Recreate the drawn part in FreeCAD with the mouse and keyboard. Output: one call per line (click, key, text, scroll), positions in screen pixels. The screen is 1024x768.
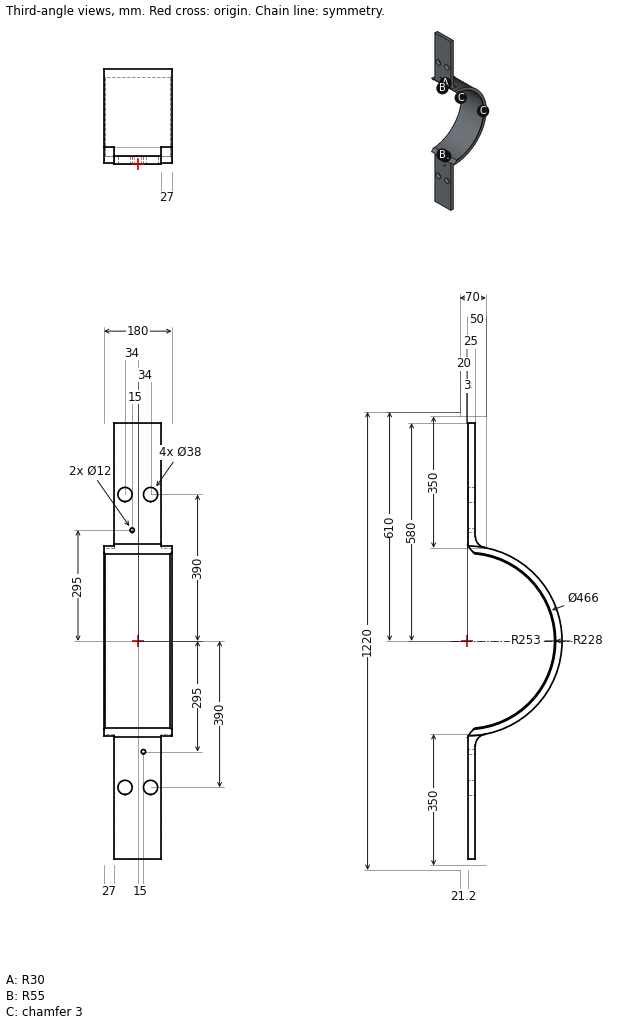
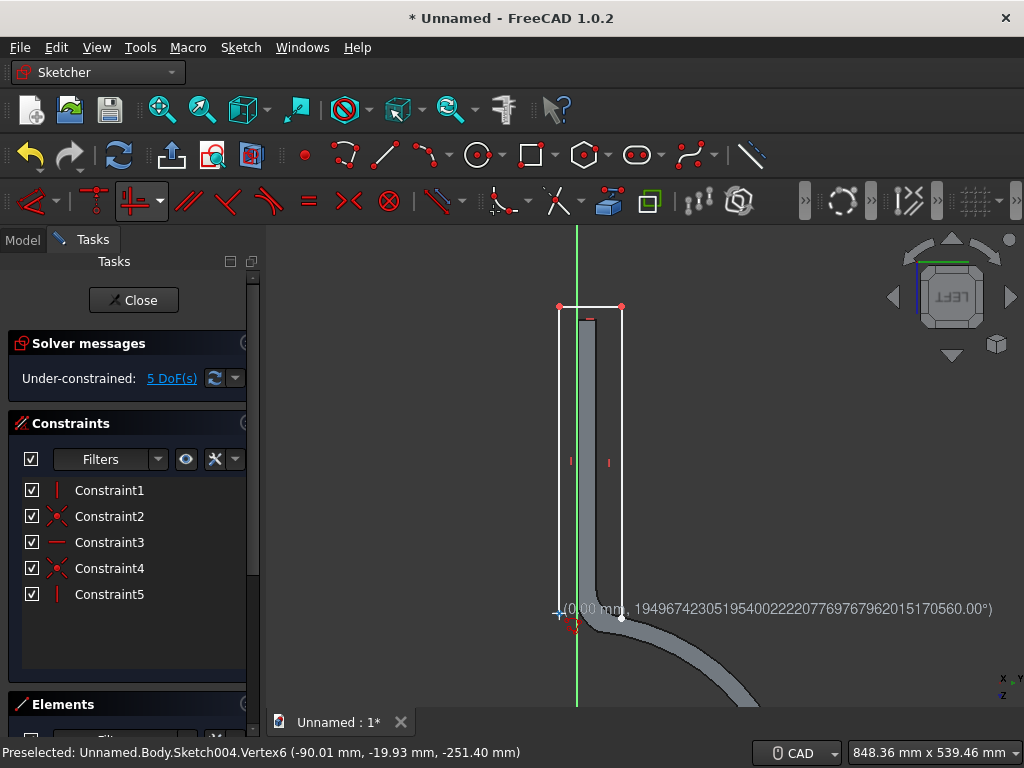
click(426, 156)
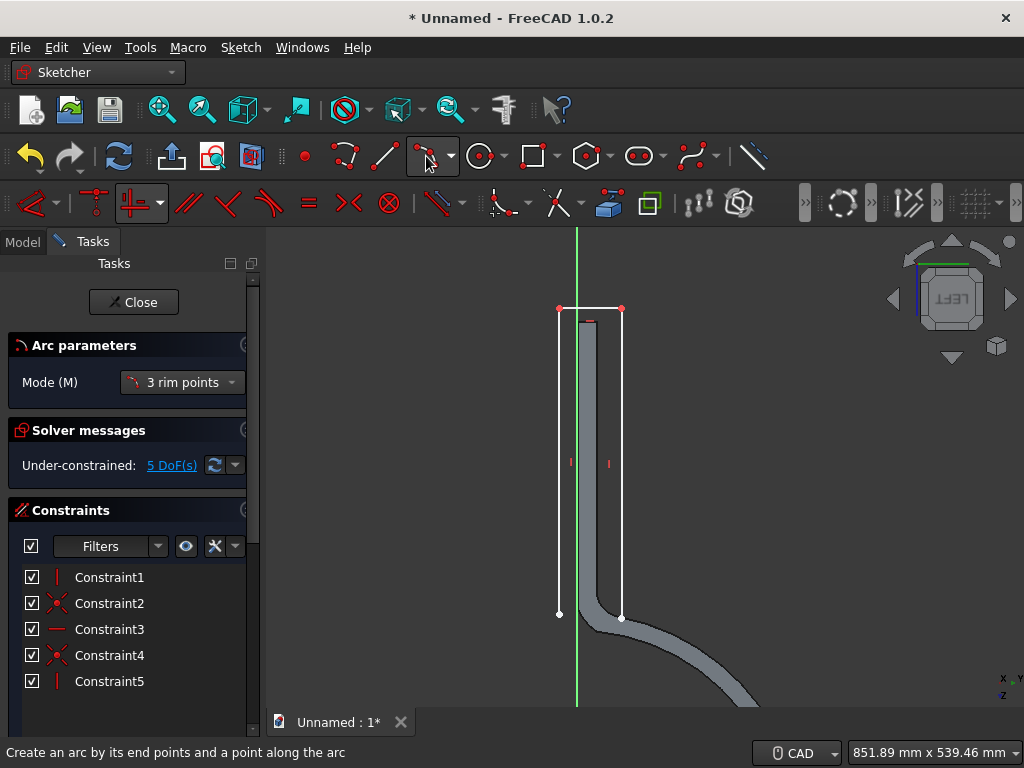
click(559, 614)
click(622, 619)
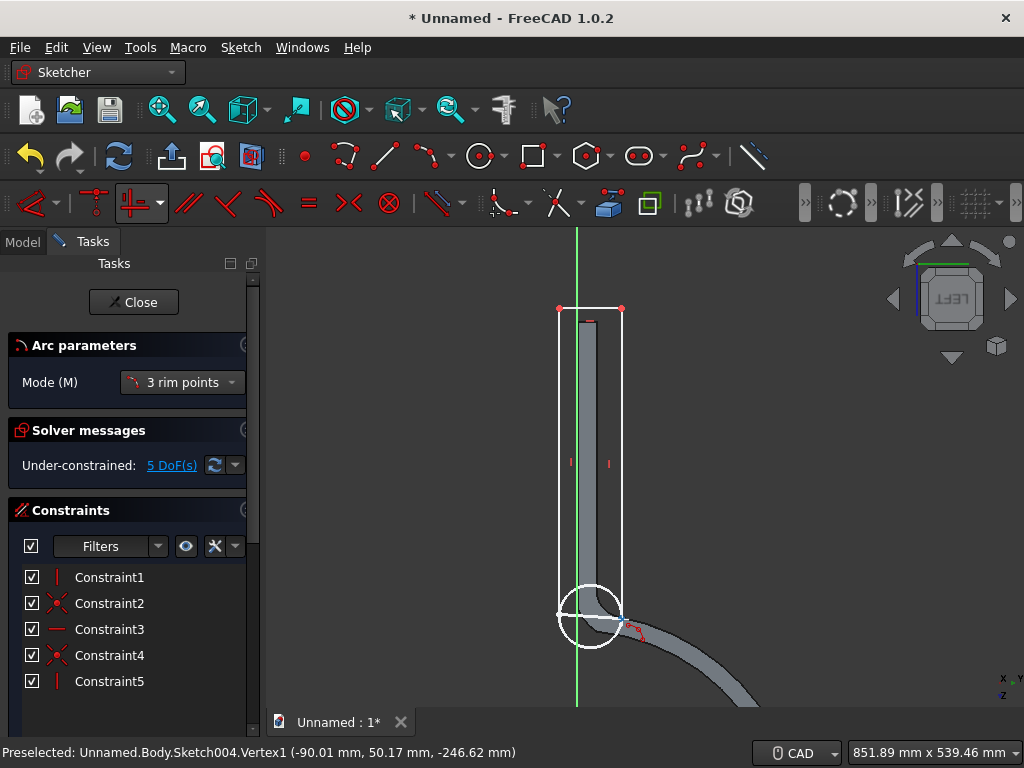
scroll(591, 613, up, 10)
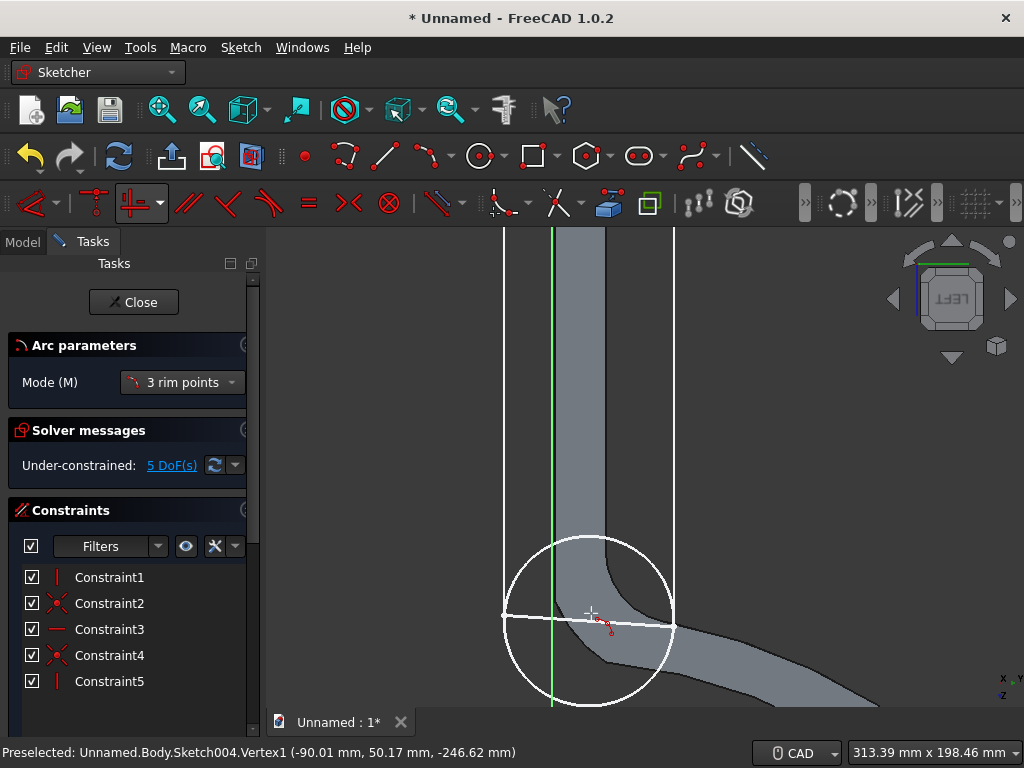
click(585, 611)
key(Escape)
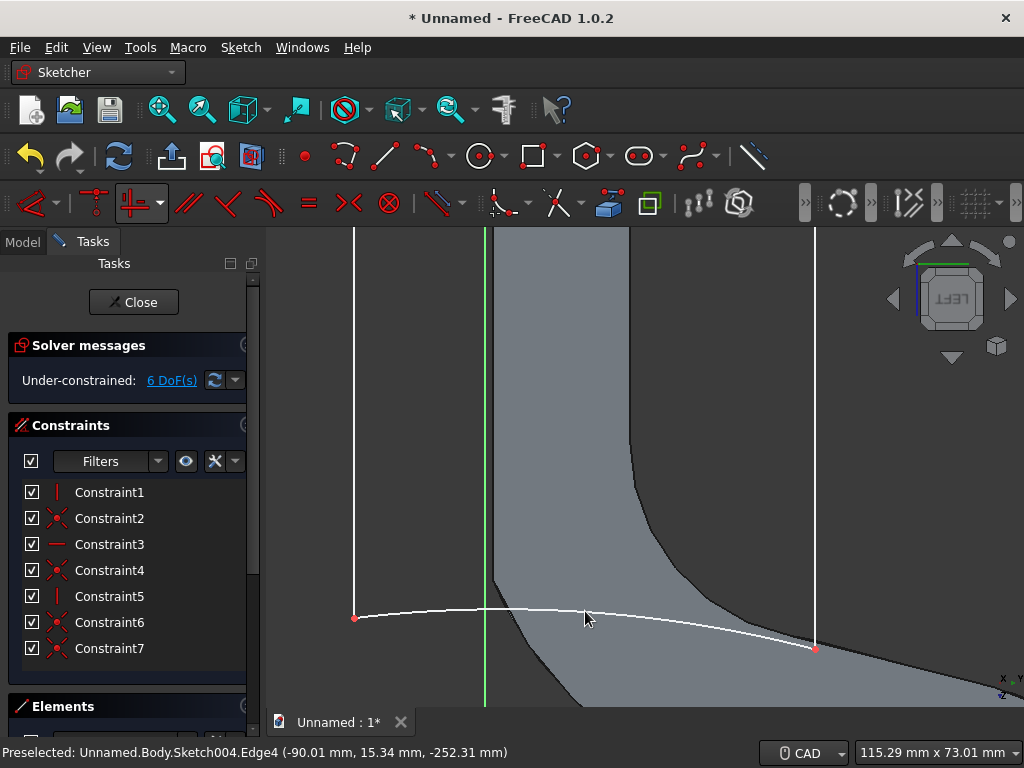
scroll(576, 480, down, 13)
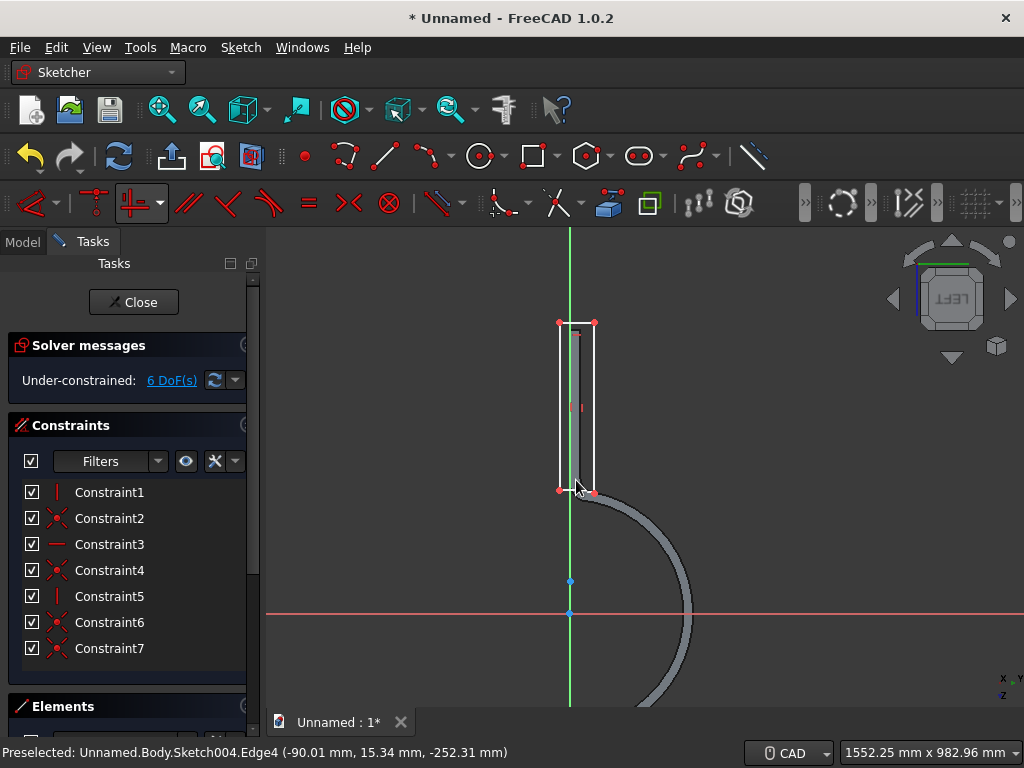
drag(560, 572, 581, 624)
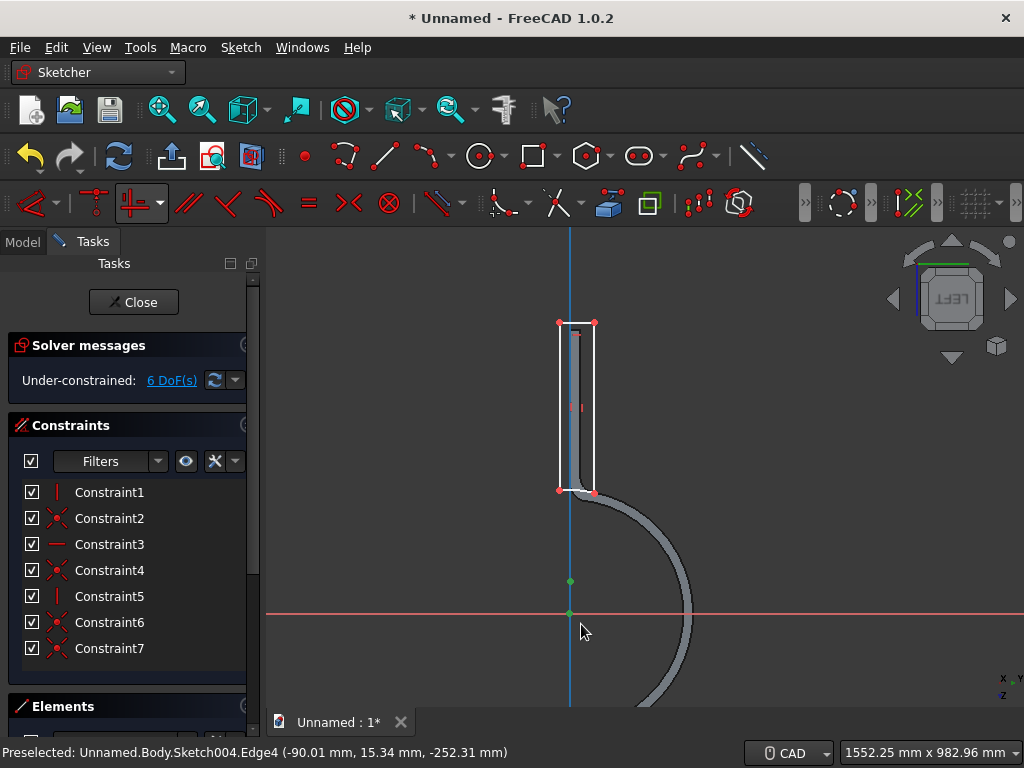
click(94, 204)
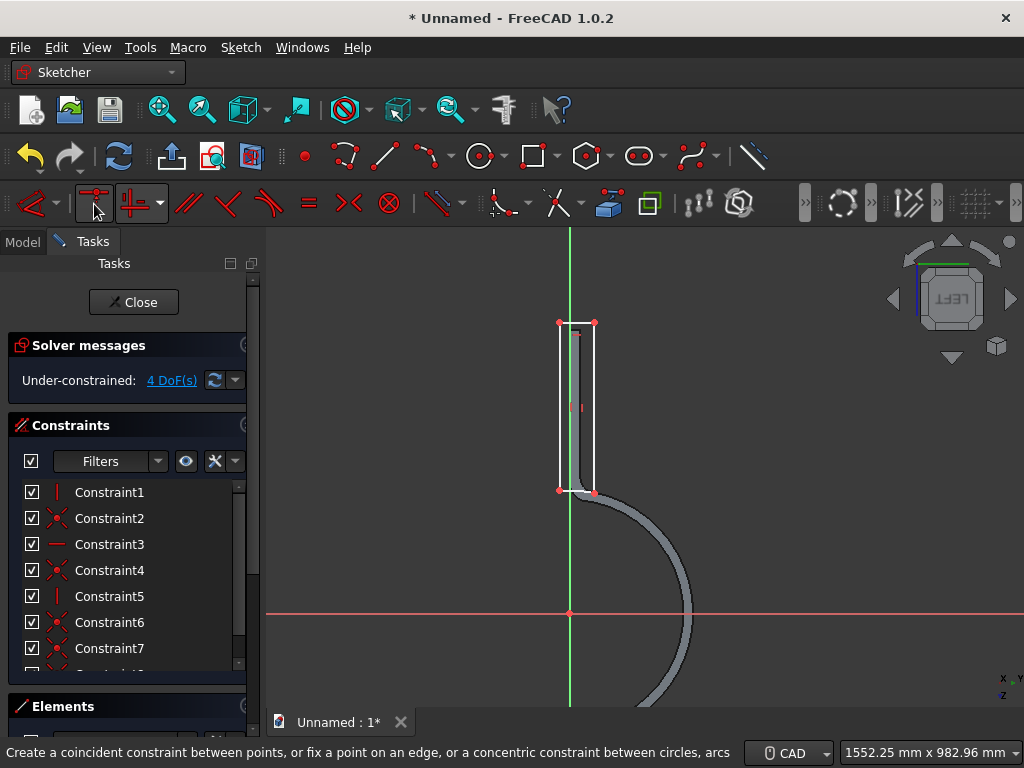
click(32, 204)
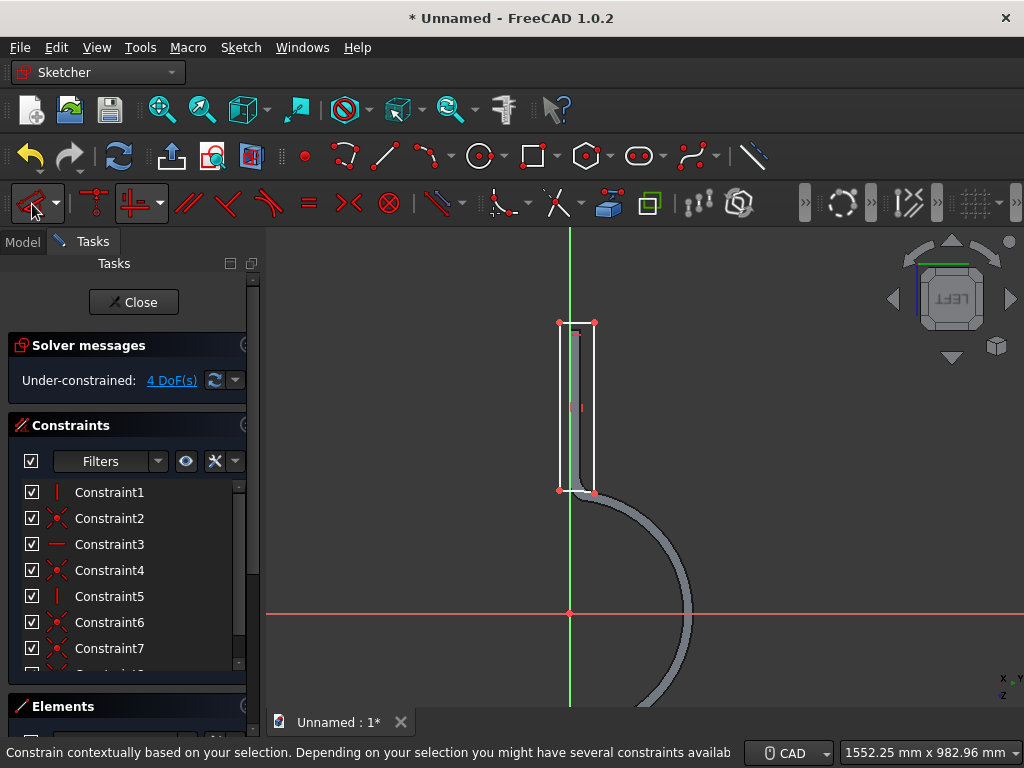
scroll(584, 491, up, 2)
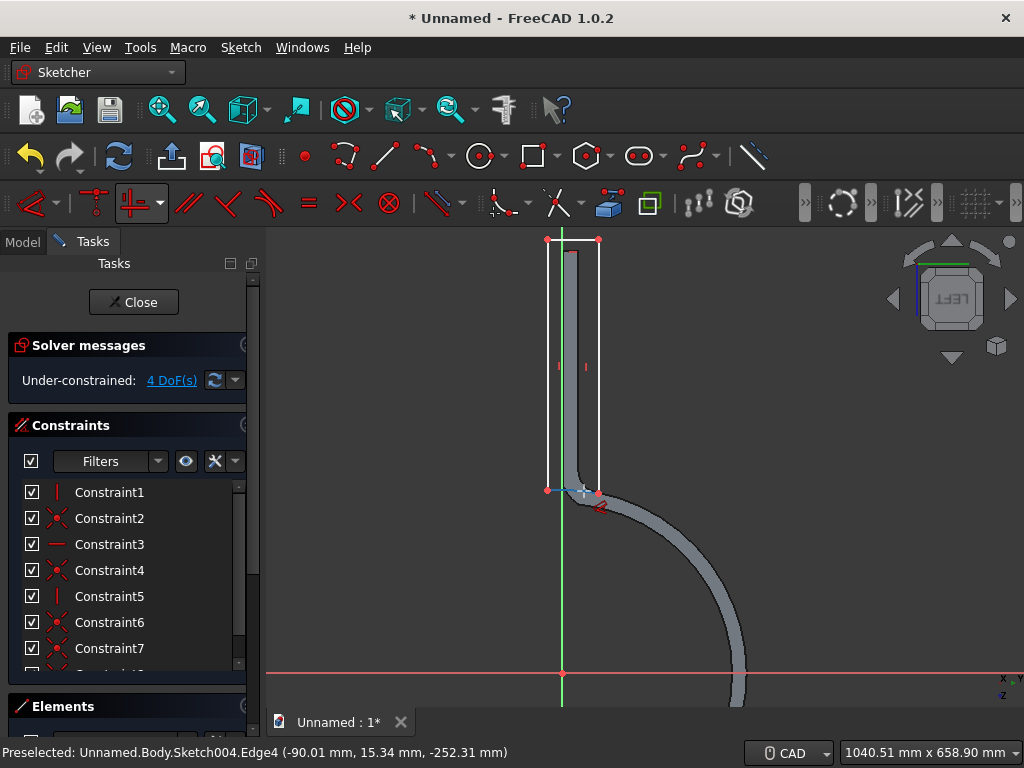
click(584, 491)
click(687, 498)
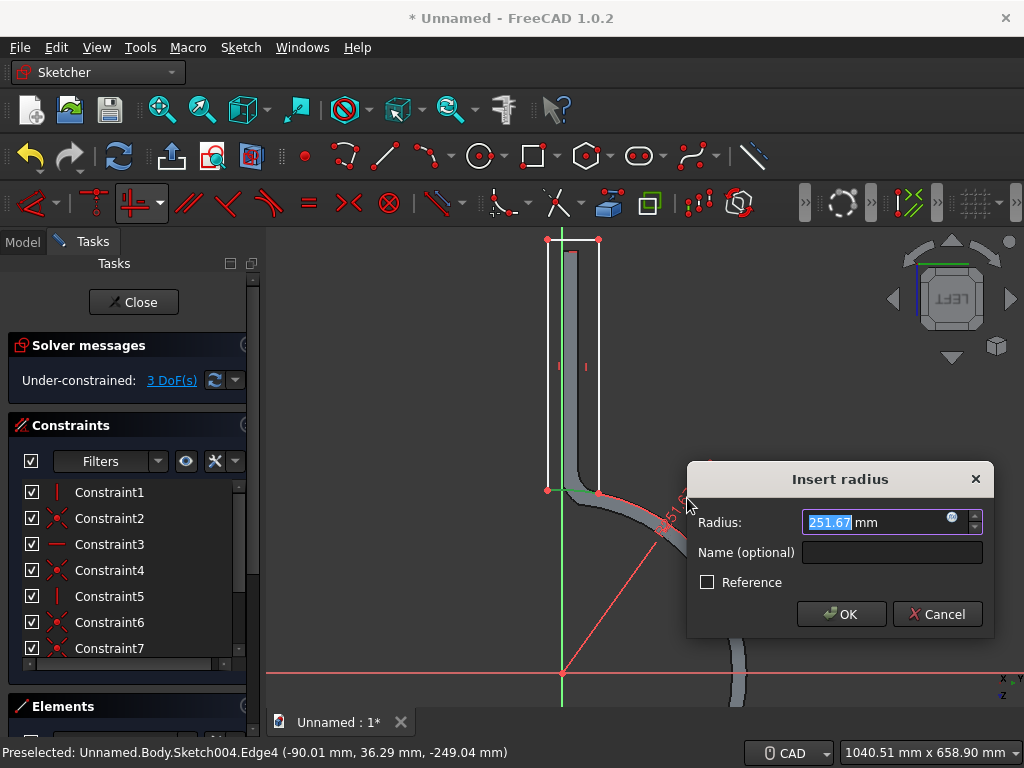
text(253)
key(Return)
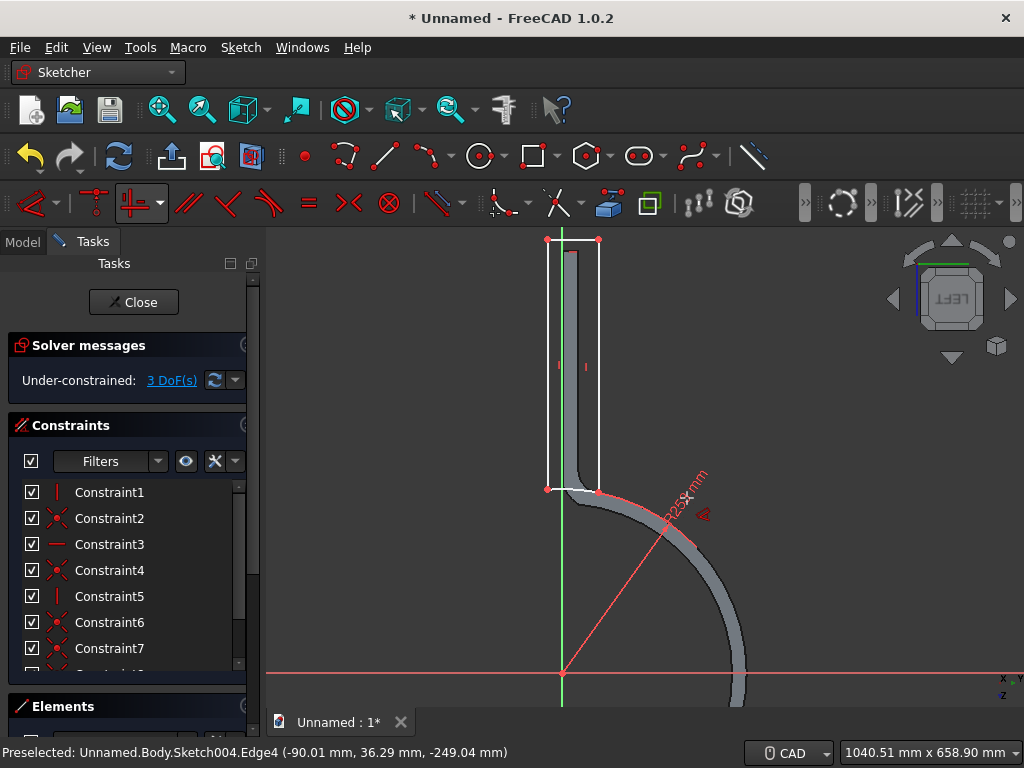
scroll(583, 490, down, 2)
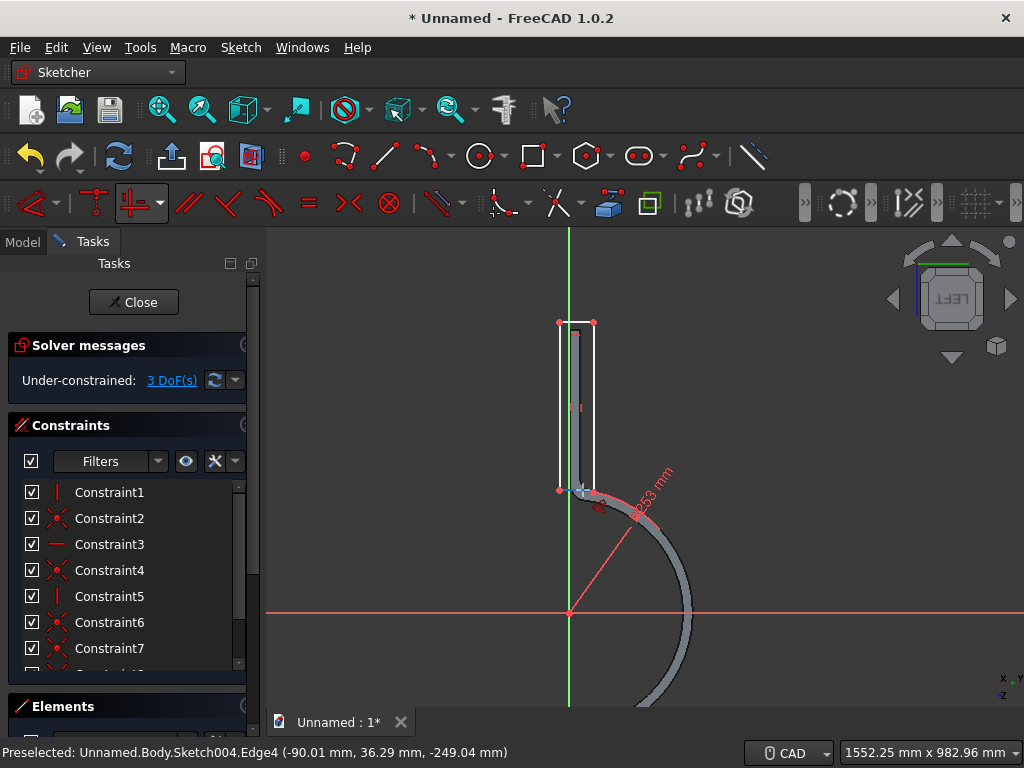
scroll(584, 322, up, 2)